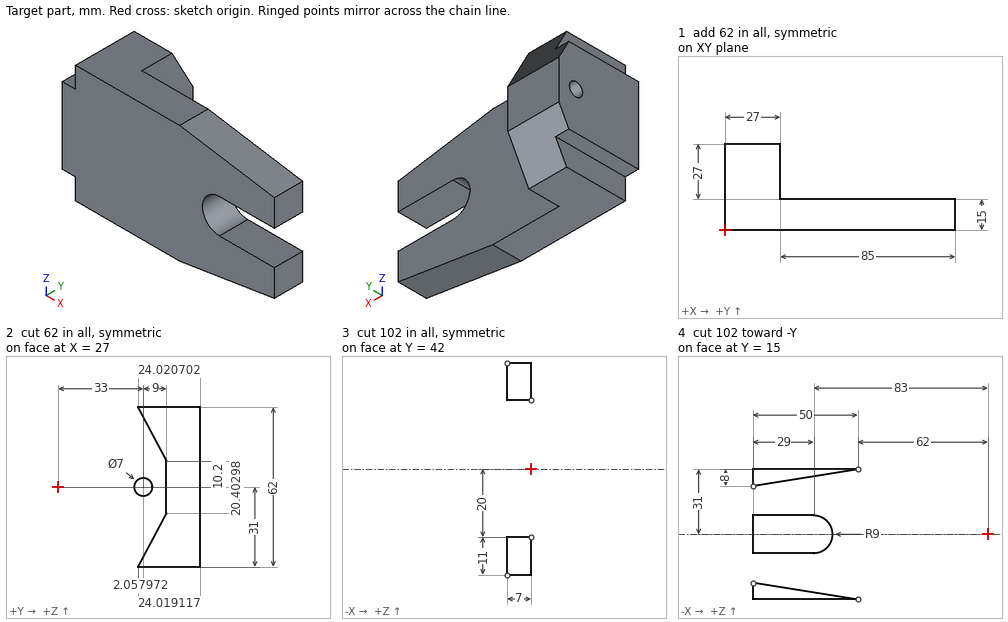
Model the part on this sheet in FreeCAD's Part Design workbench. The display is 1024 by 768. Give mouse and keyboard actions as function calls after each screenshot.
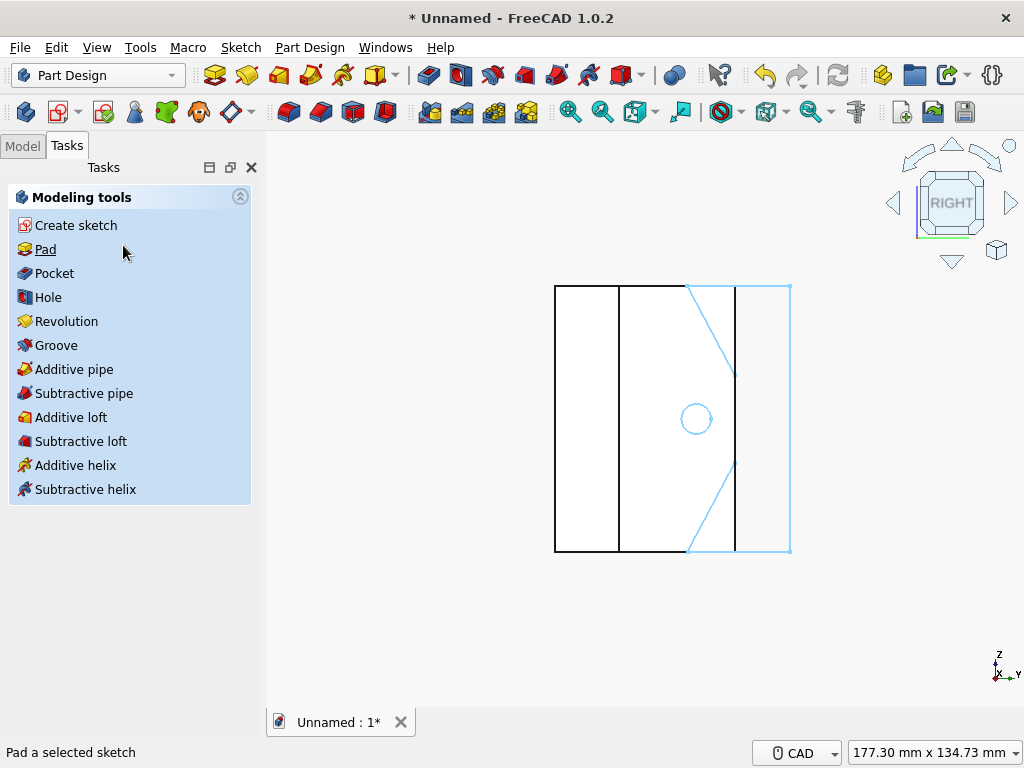
click(430, 76)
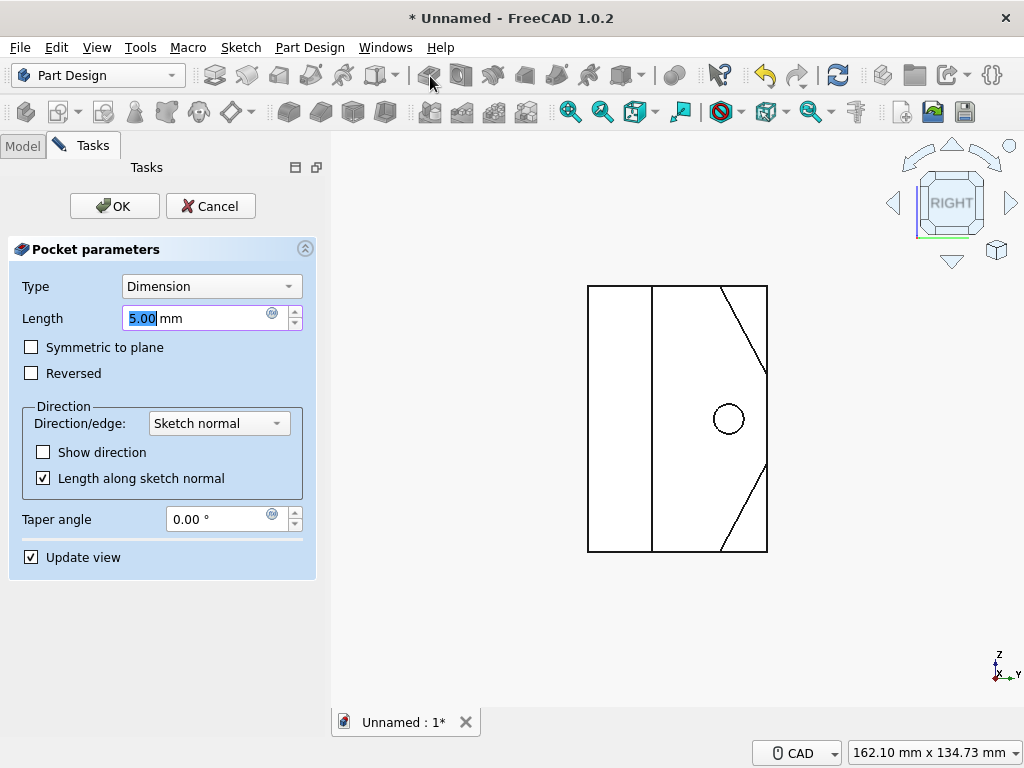
text(62)
key(Tab)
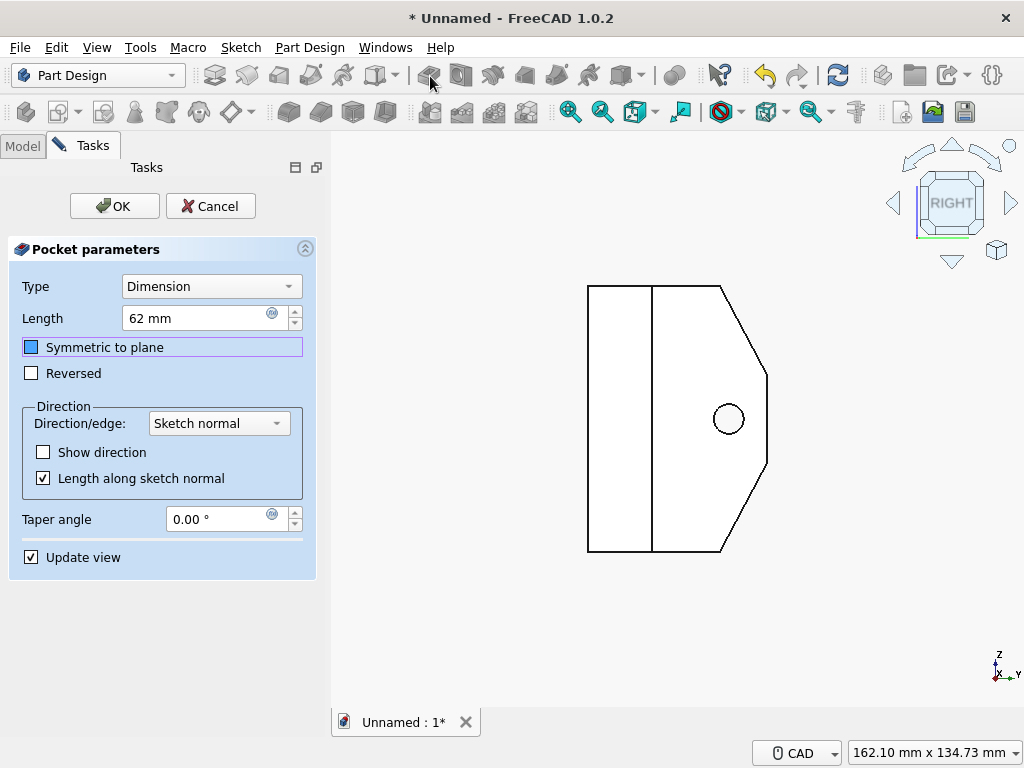
click(30, 347)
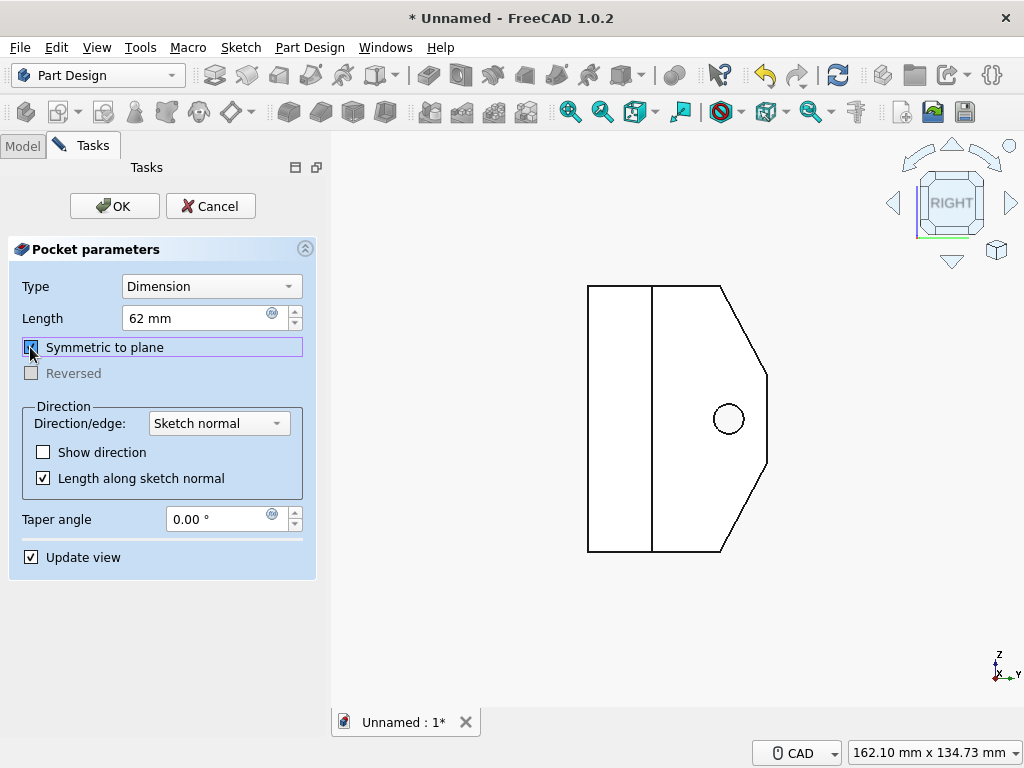
click(115, 206)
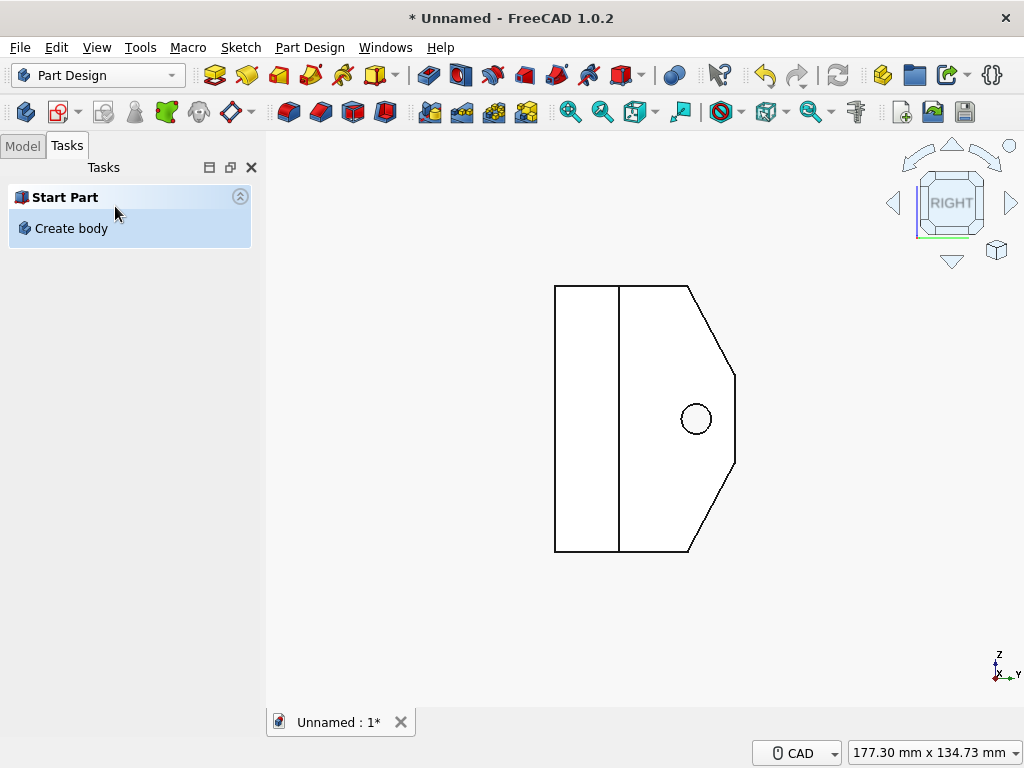
key(4)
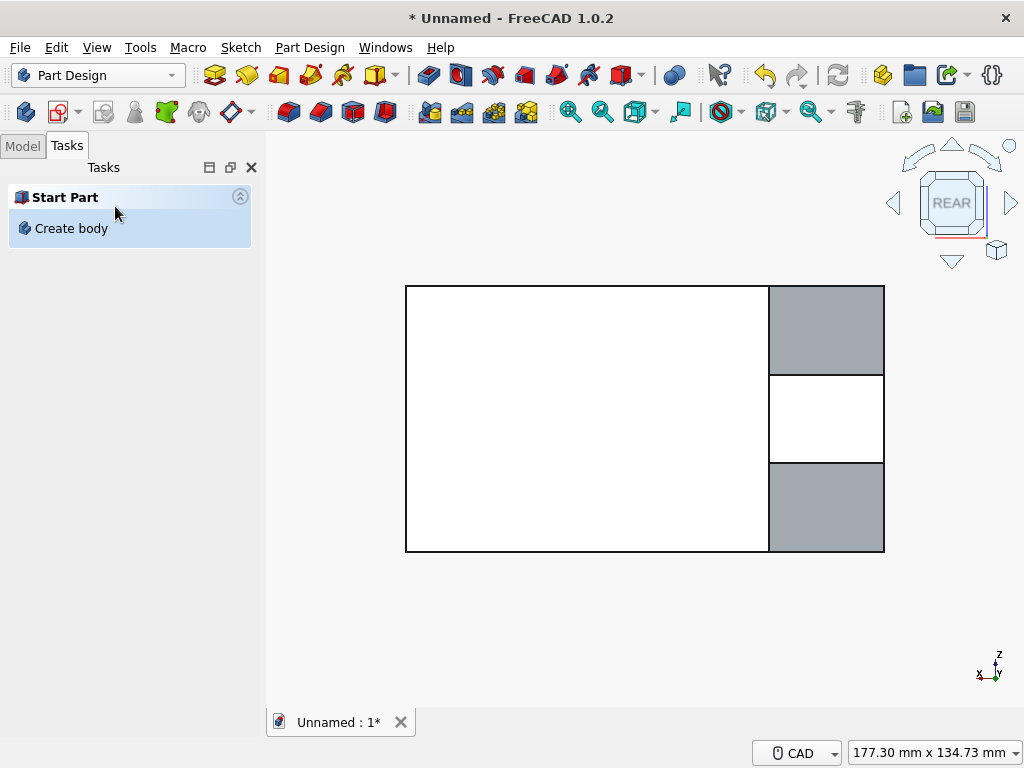
click(827, 418)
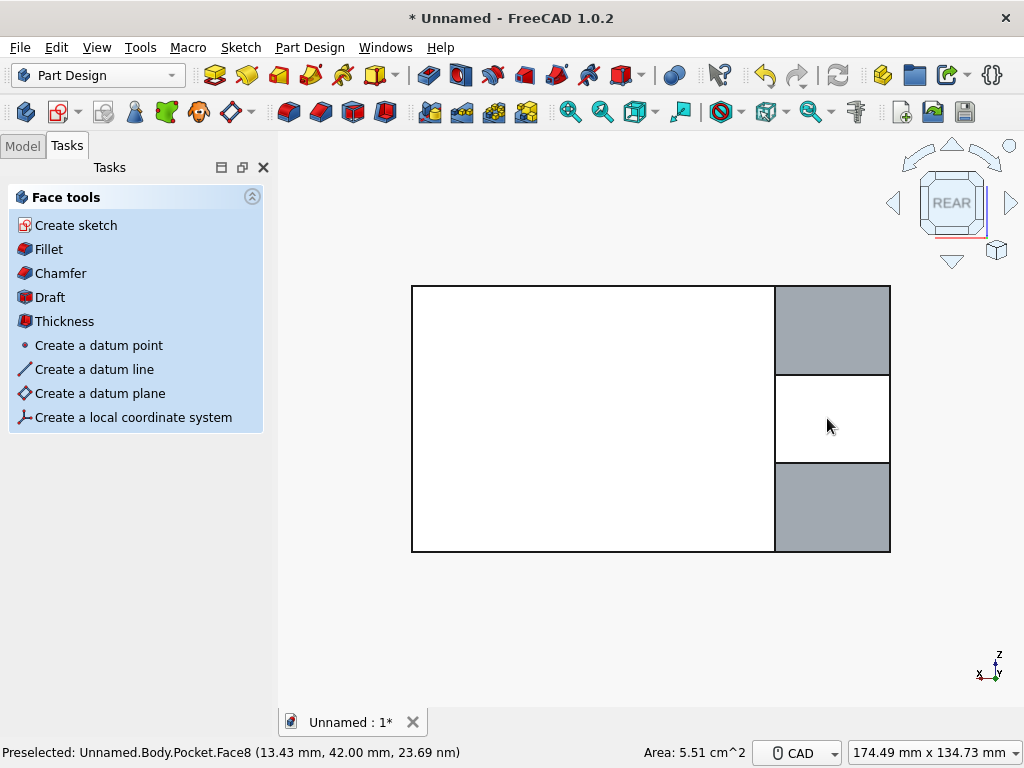
click(58, 112)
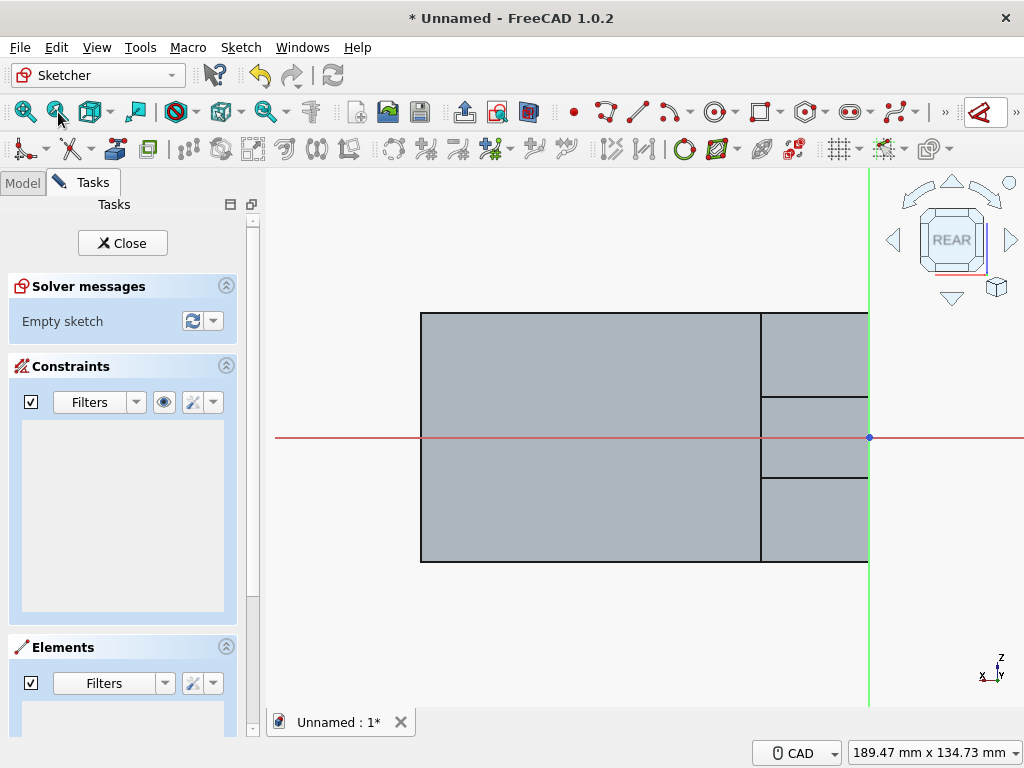
scroll(294, 437, down, 1)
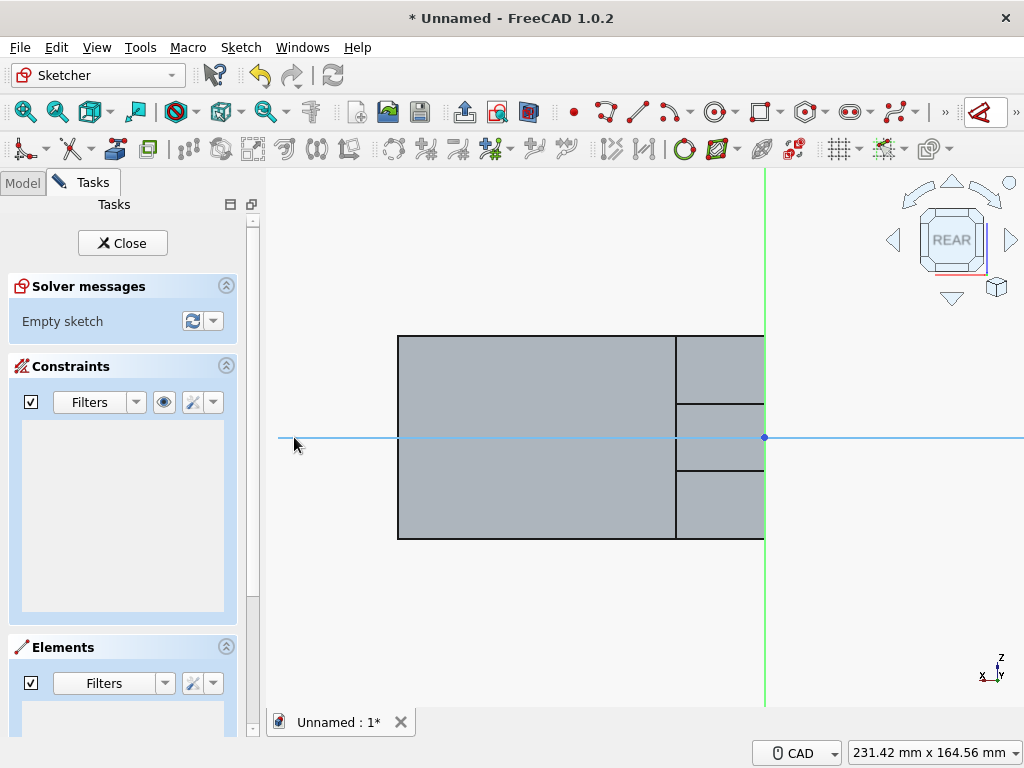
scroll(859, 438, up, 3)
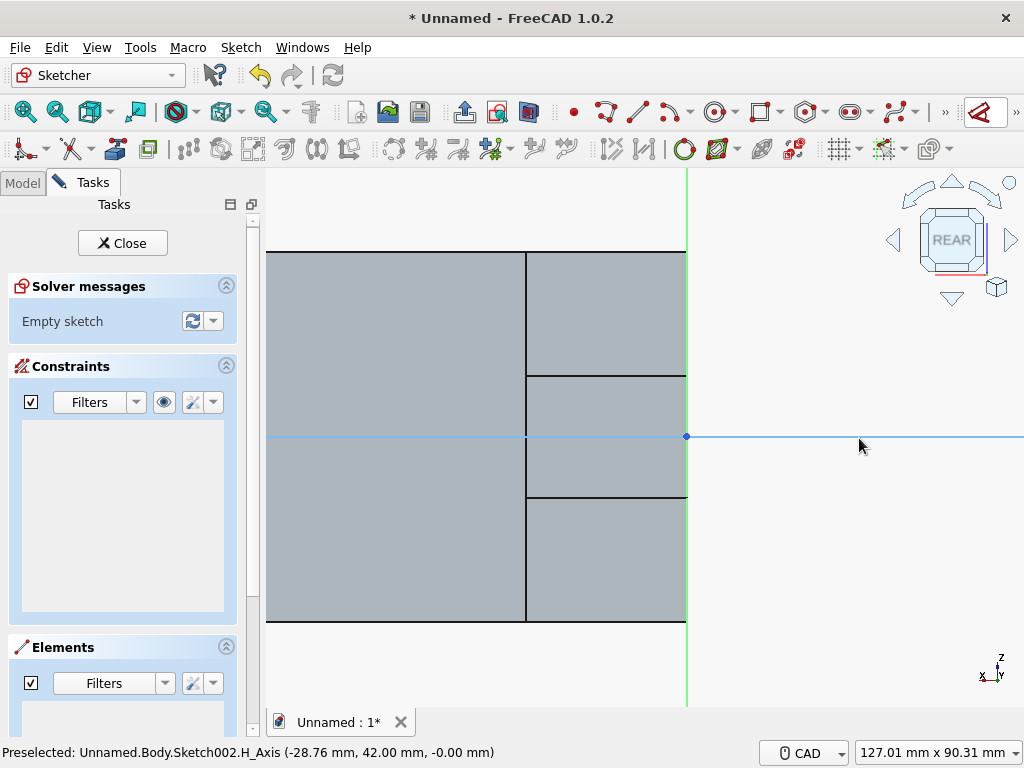
click(760, 112)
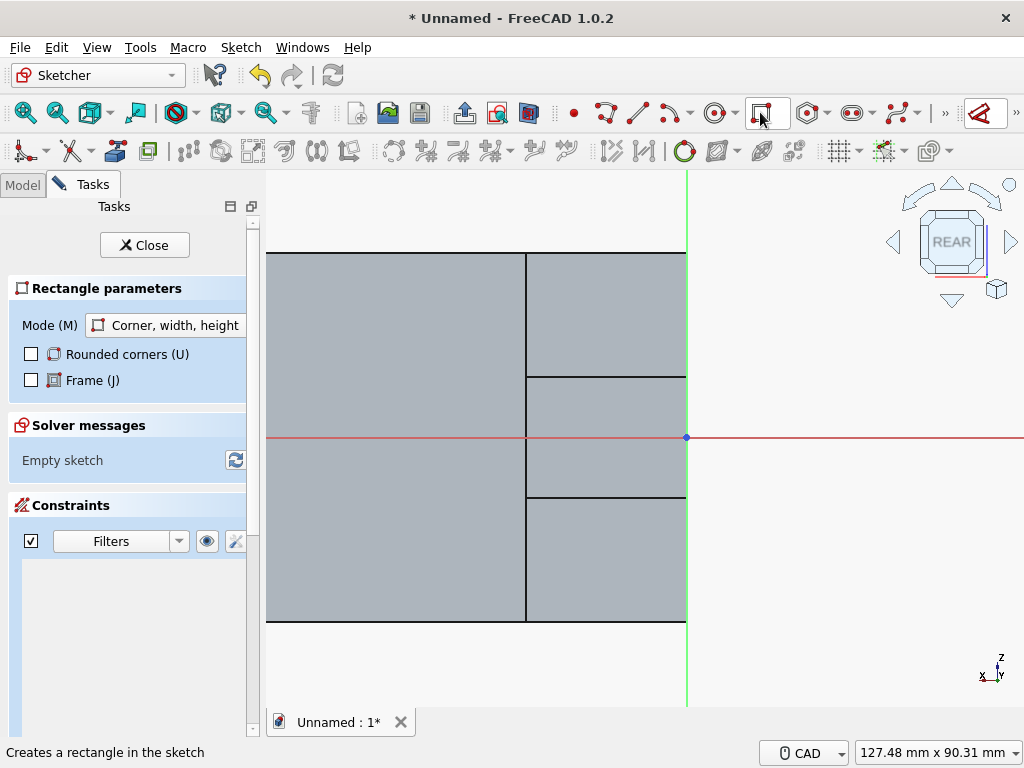
click(645, 557)
click(687, 622)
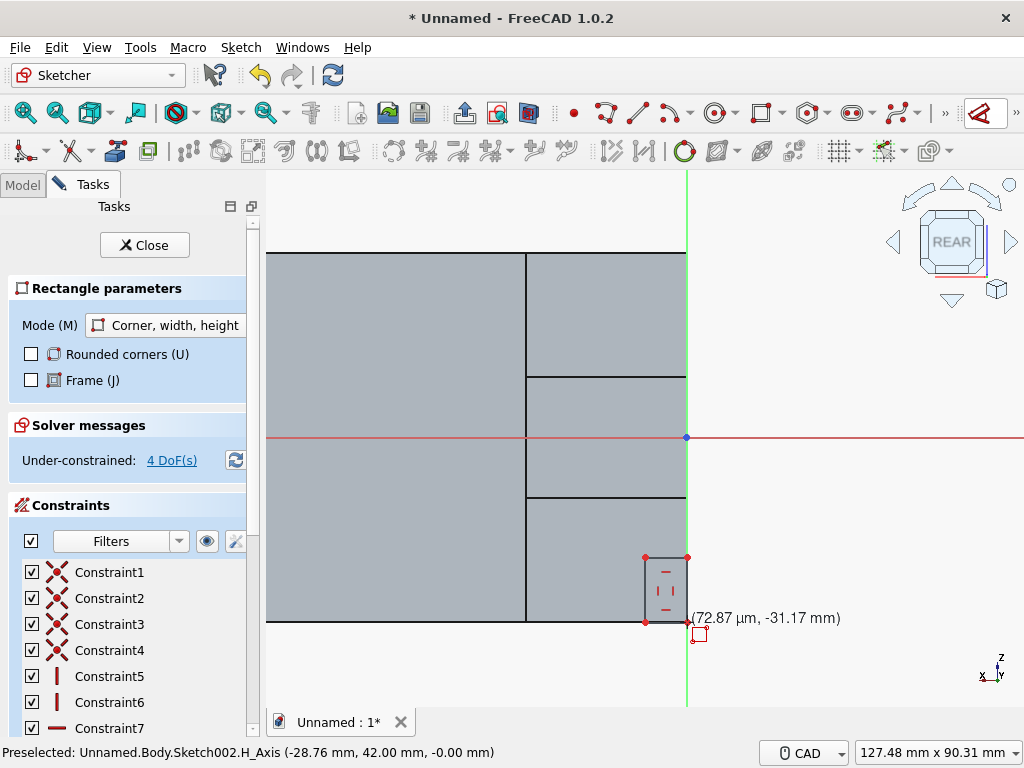
click(645, 253)
click(687, 319)
key(Escape)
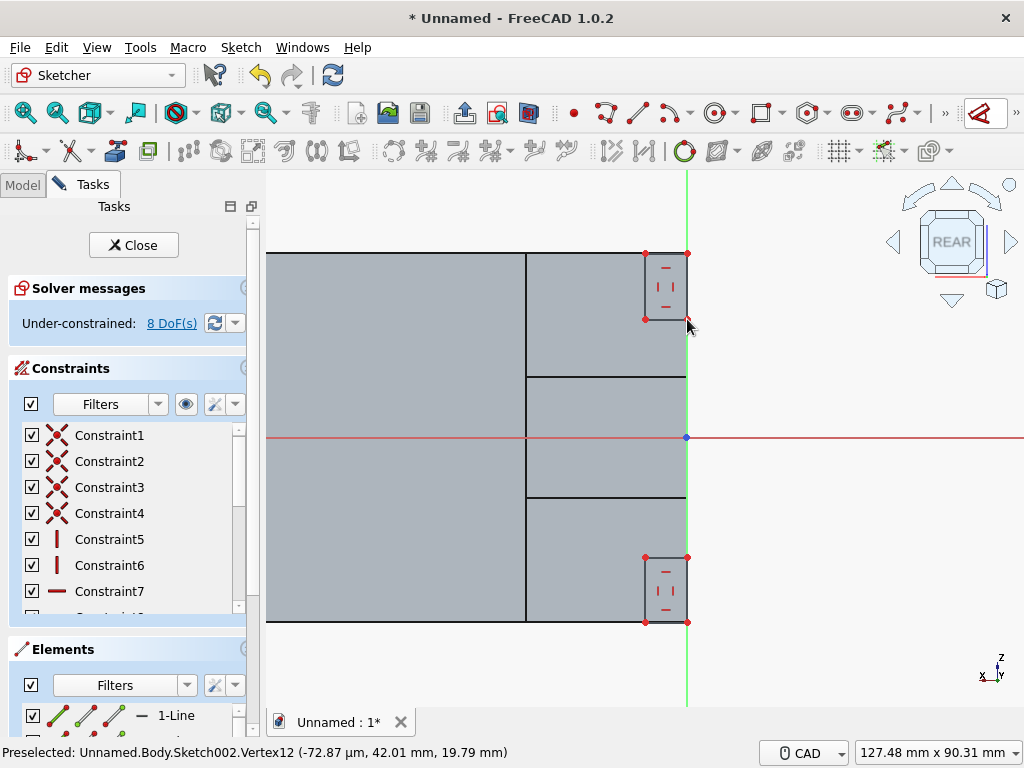
click(645, 623)